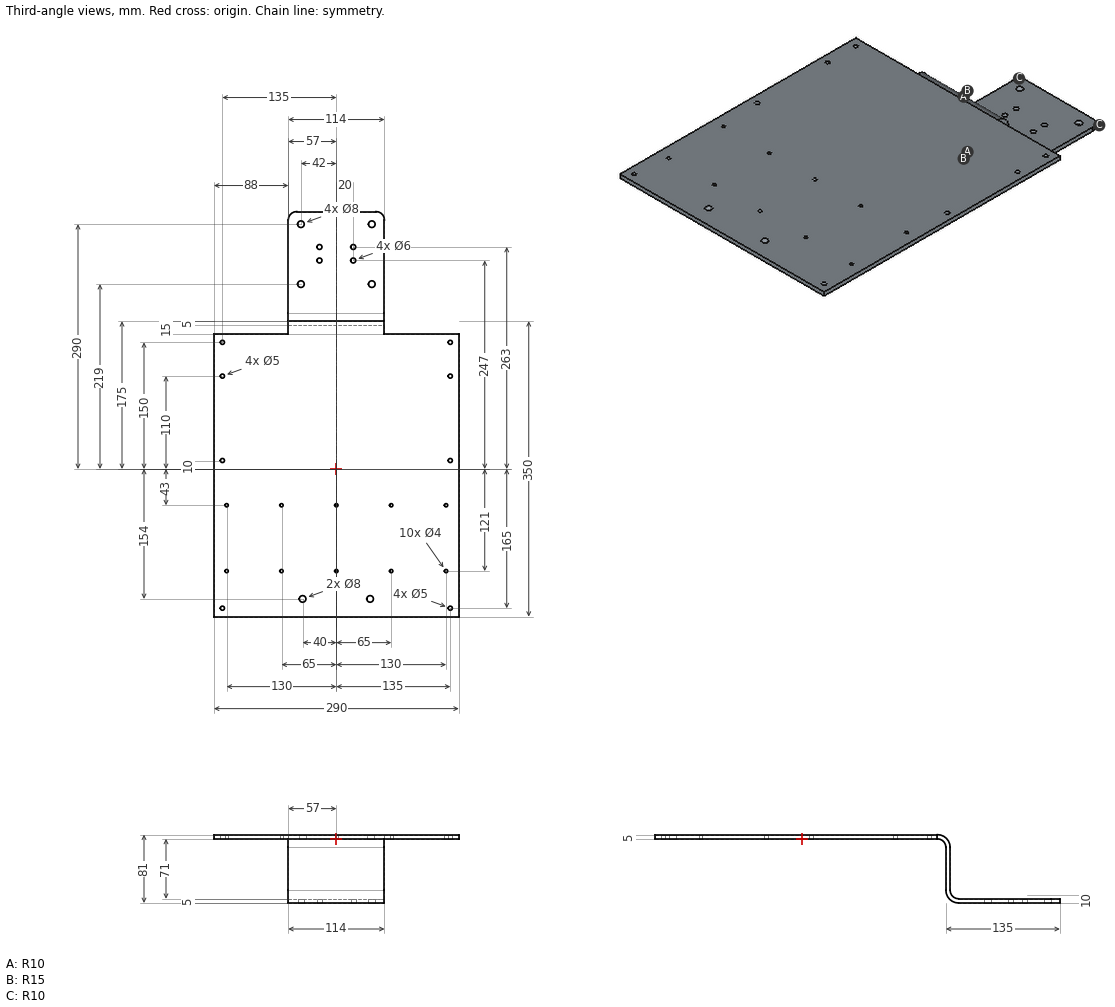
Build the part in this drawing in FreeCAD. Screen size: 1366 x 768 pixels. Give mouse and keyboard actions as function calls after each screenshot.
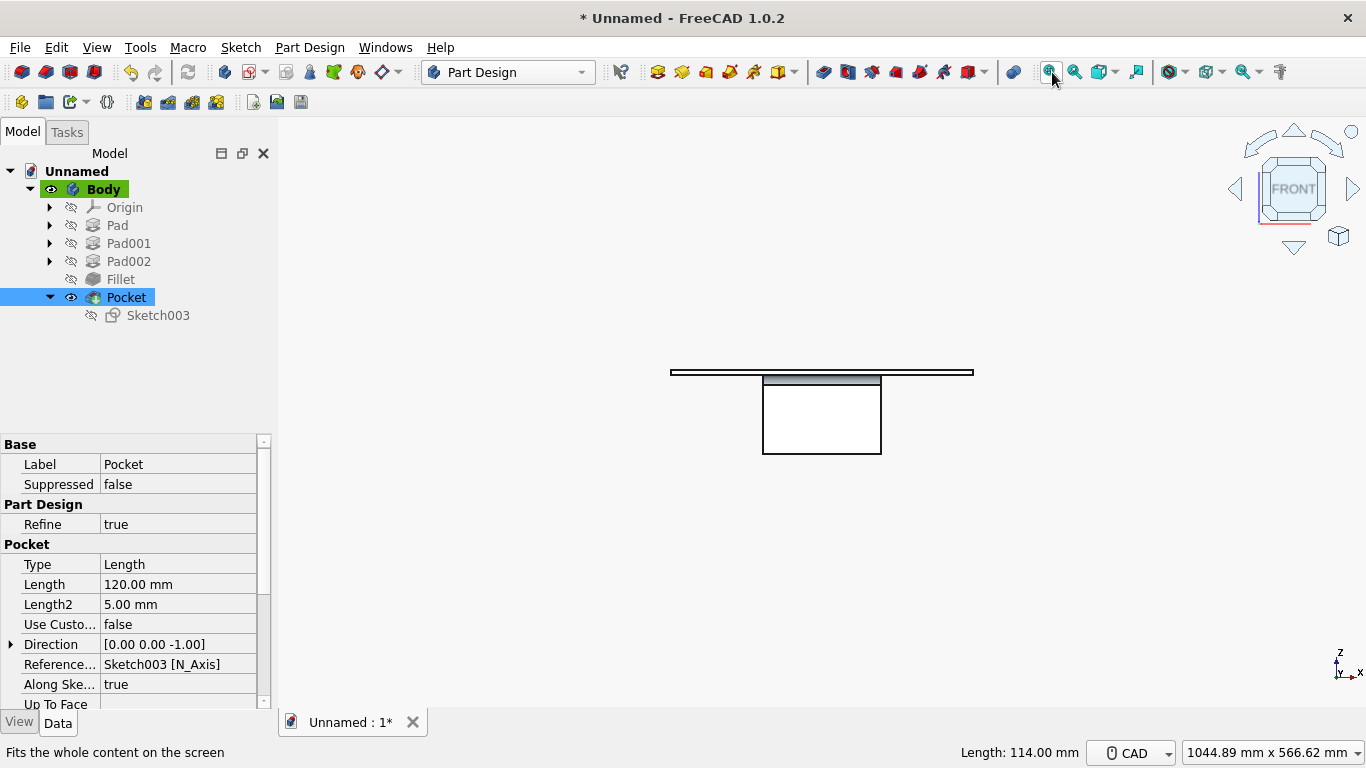
click(822, 453, ctrl)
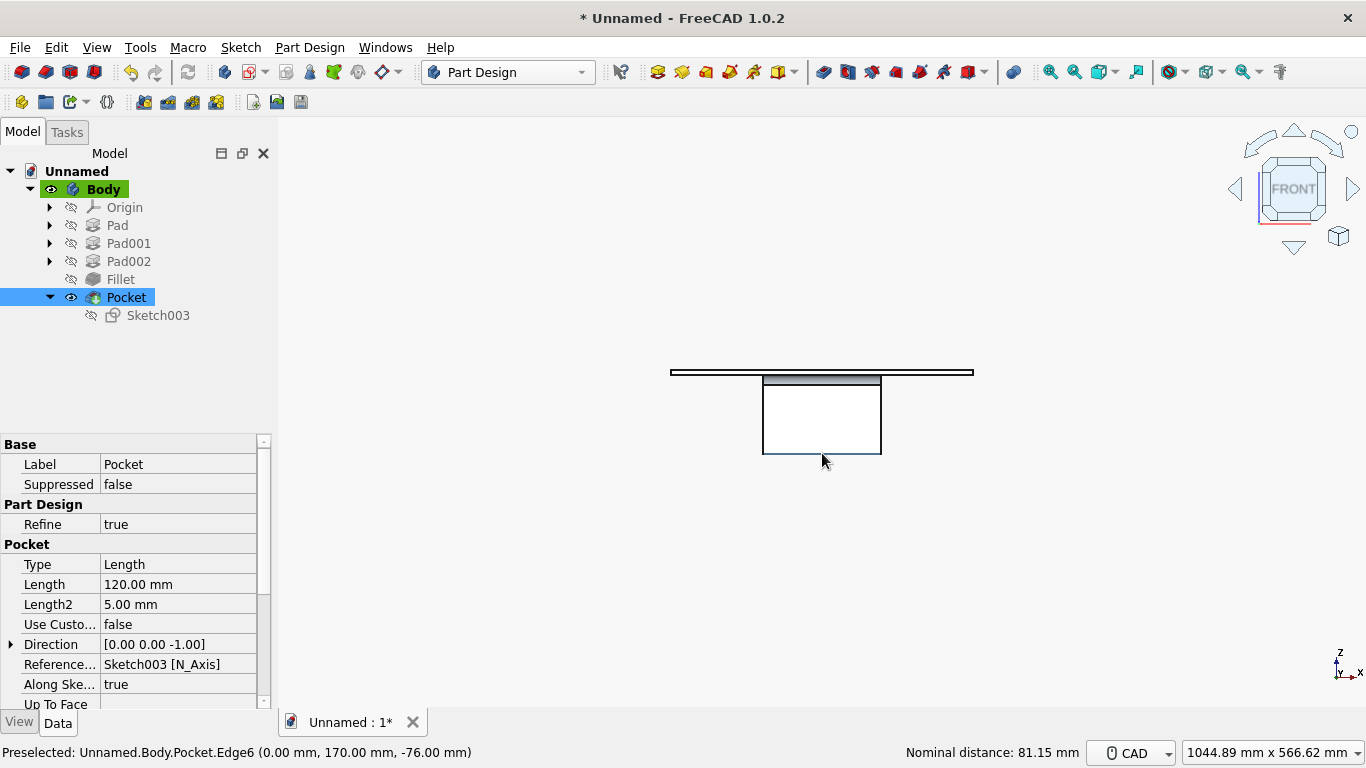
click(22, 72)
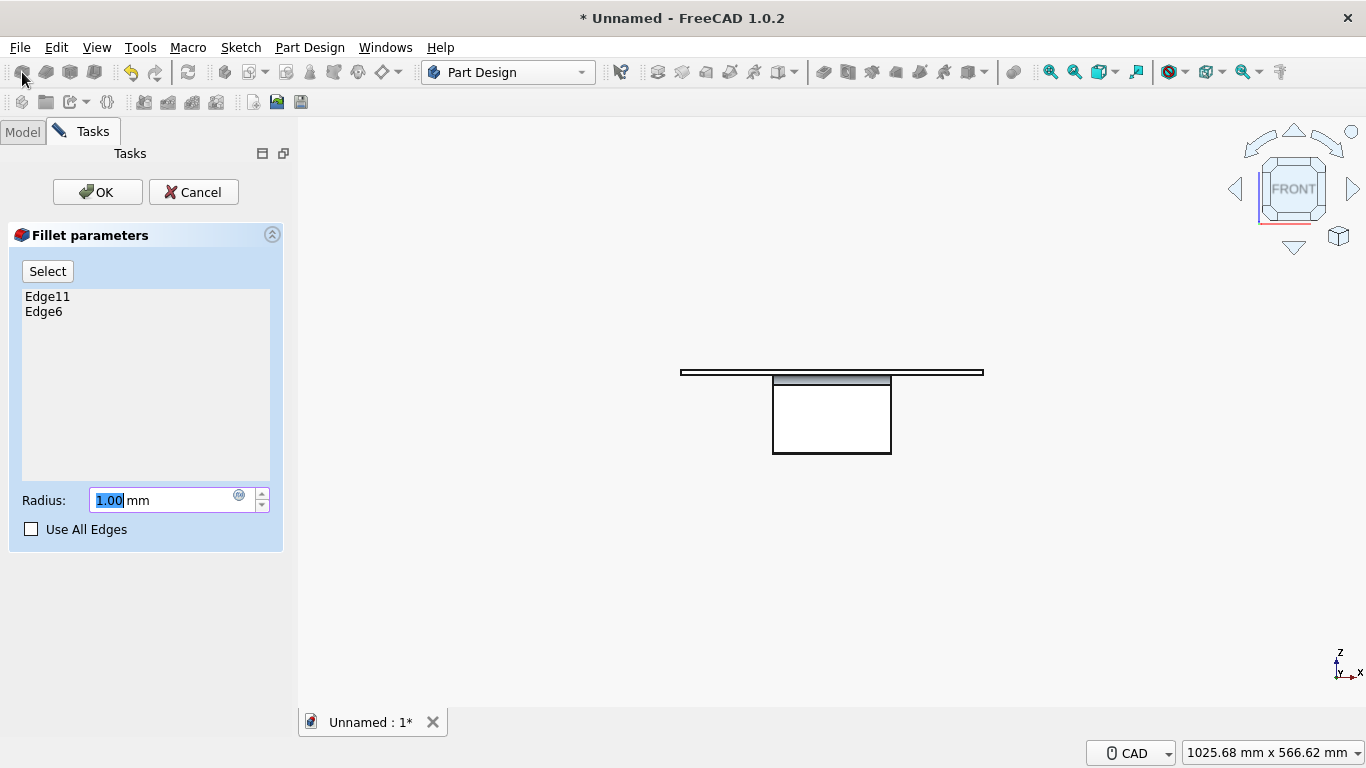
text(15)
key(Tab)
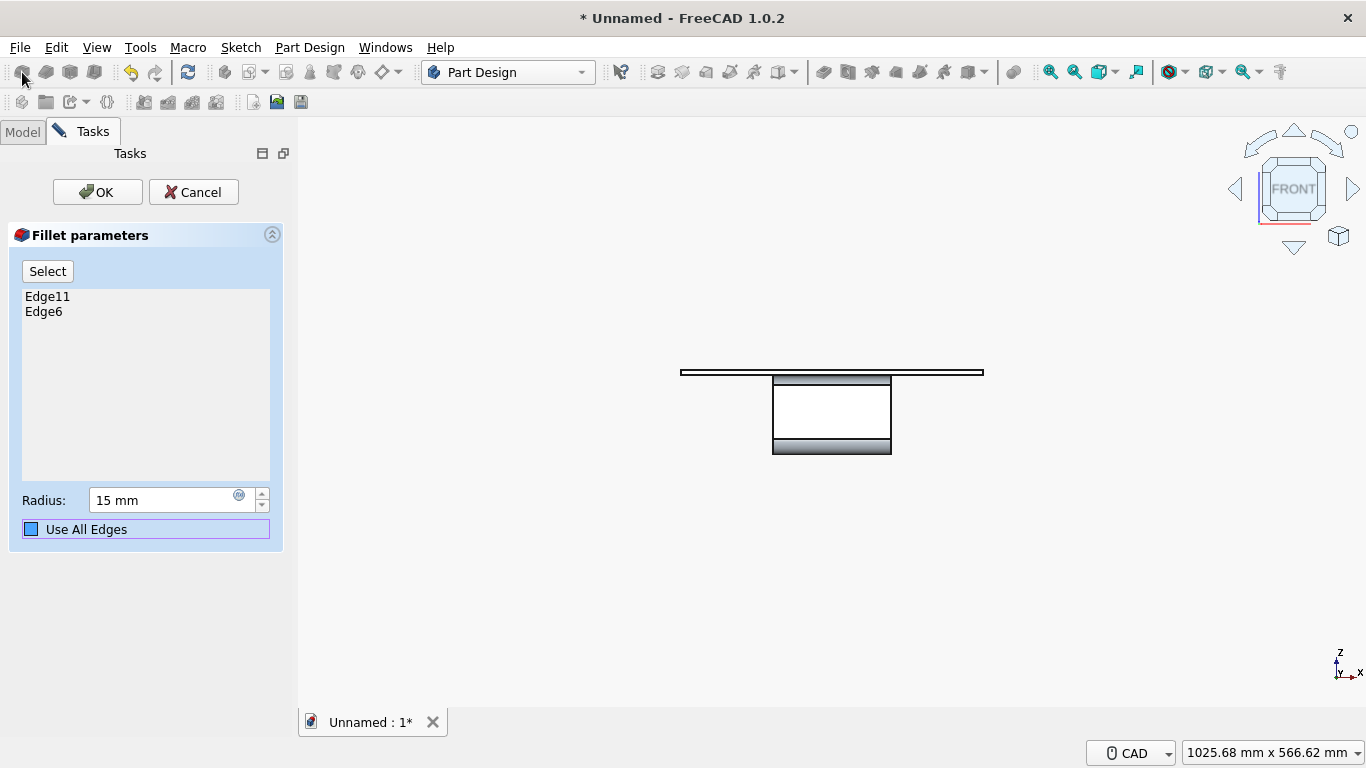
click(98, 192)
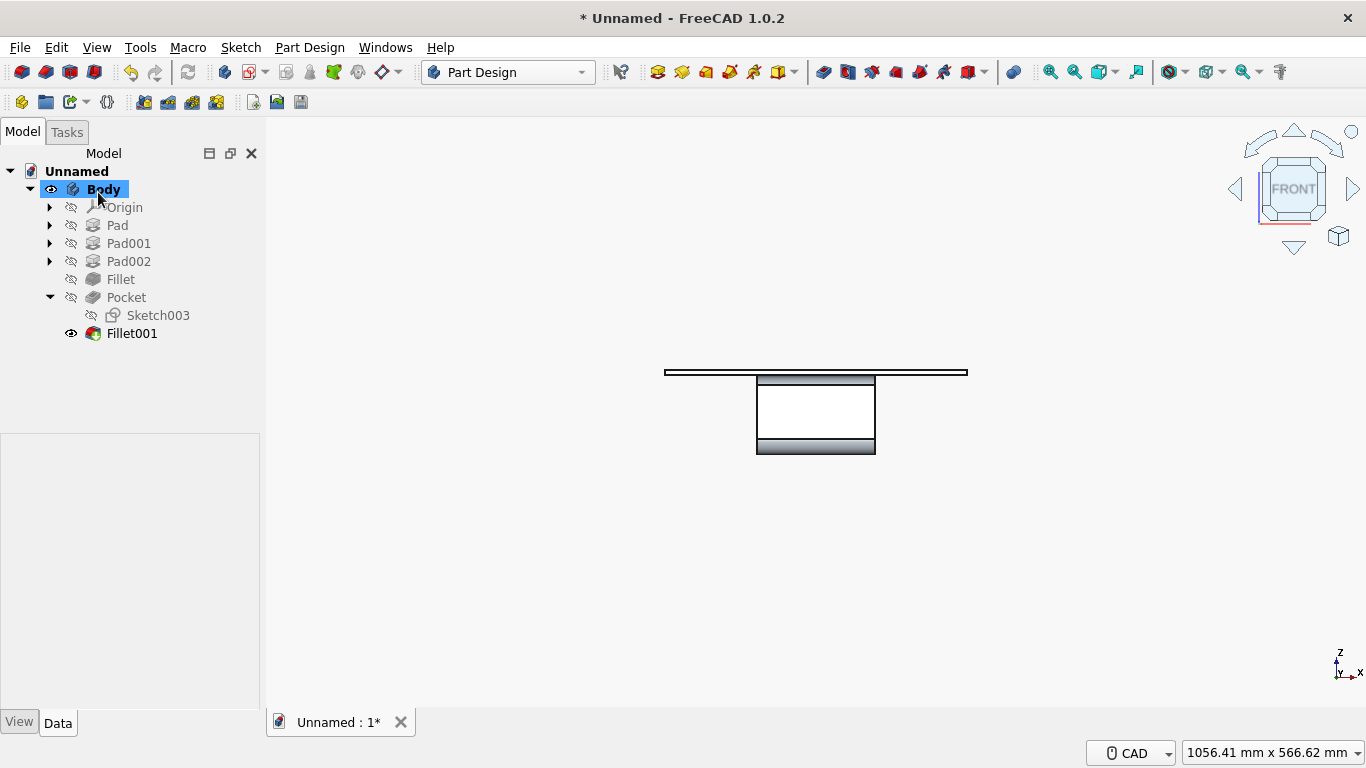
click(1052, 72)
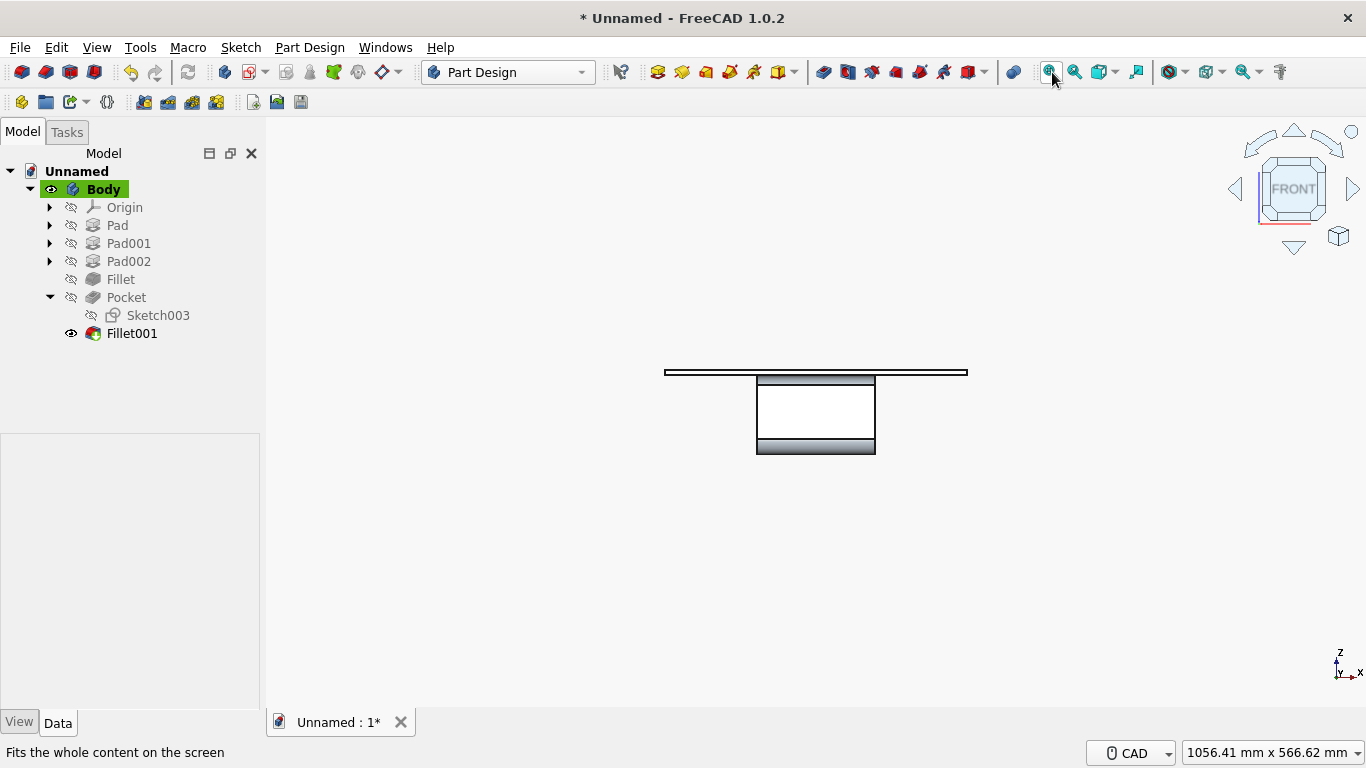
scroll(875, 451, up, 11)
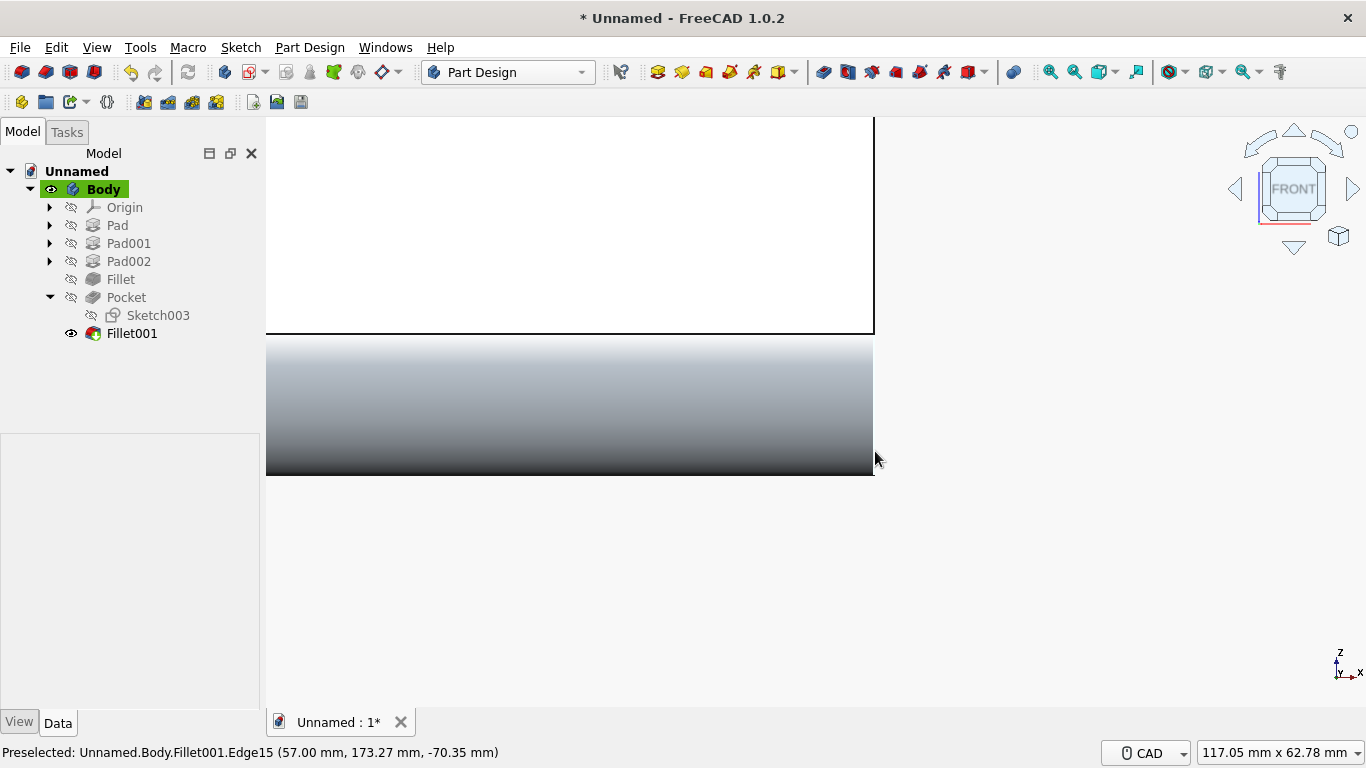
click(1052, 72)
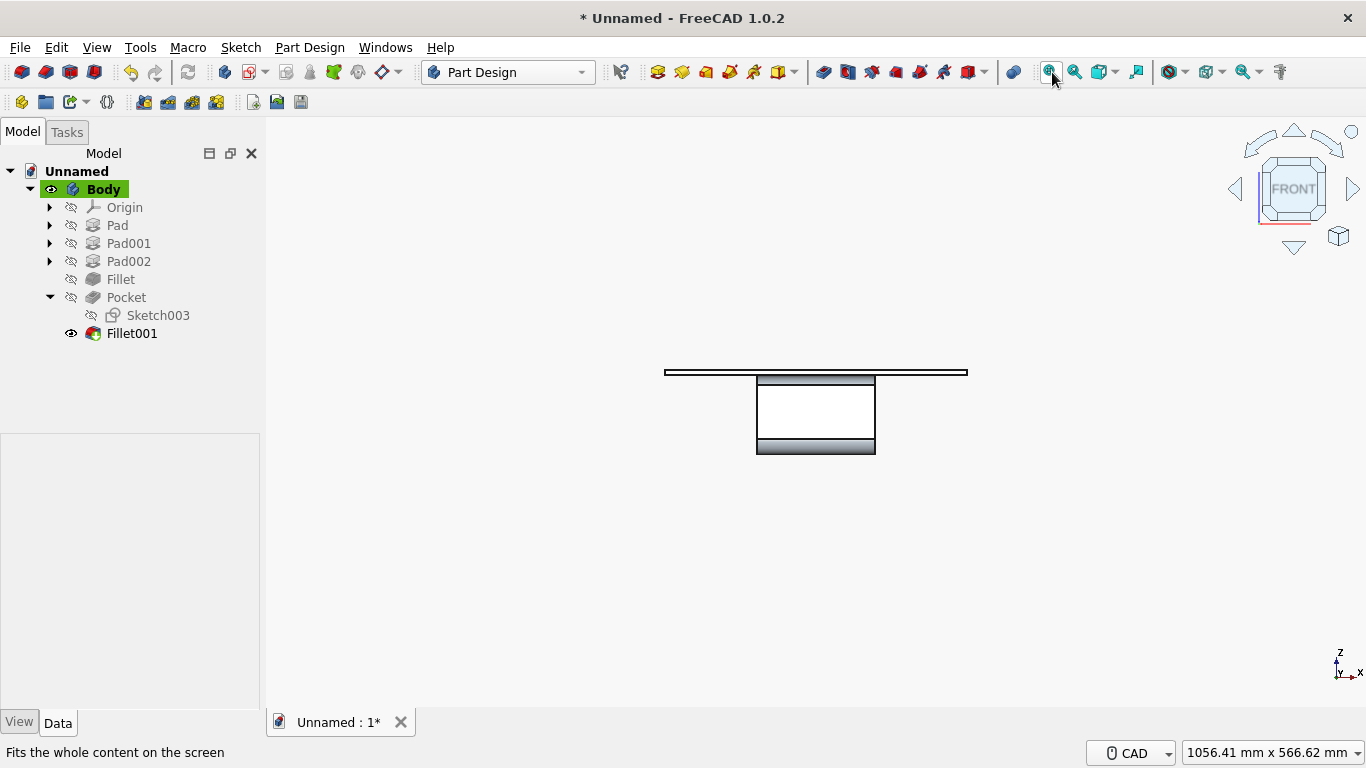
key(0)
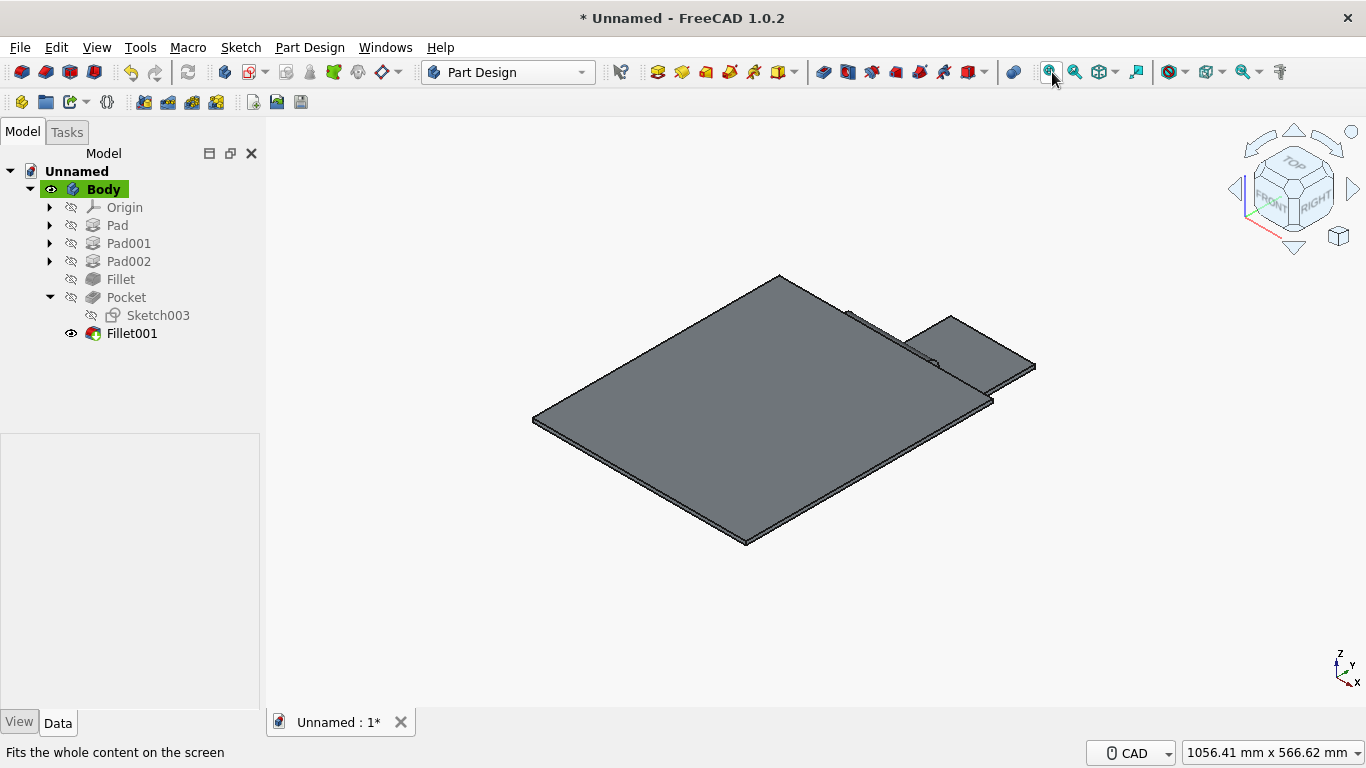
scroll(1035, 366, up, 11)